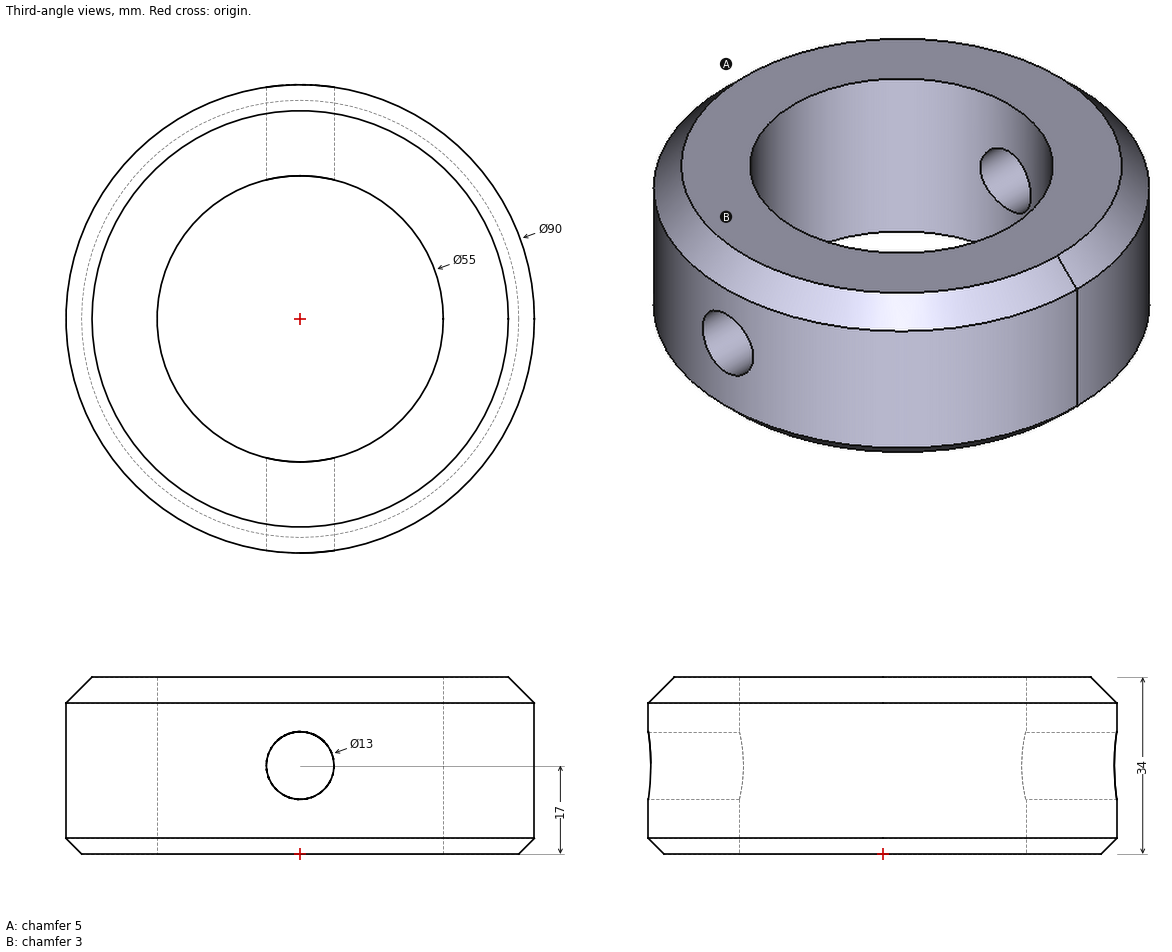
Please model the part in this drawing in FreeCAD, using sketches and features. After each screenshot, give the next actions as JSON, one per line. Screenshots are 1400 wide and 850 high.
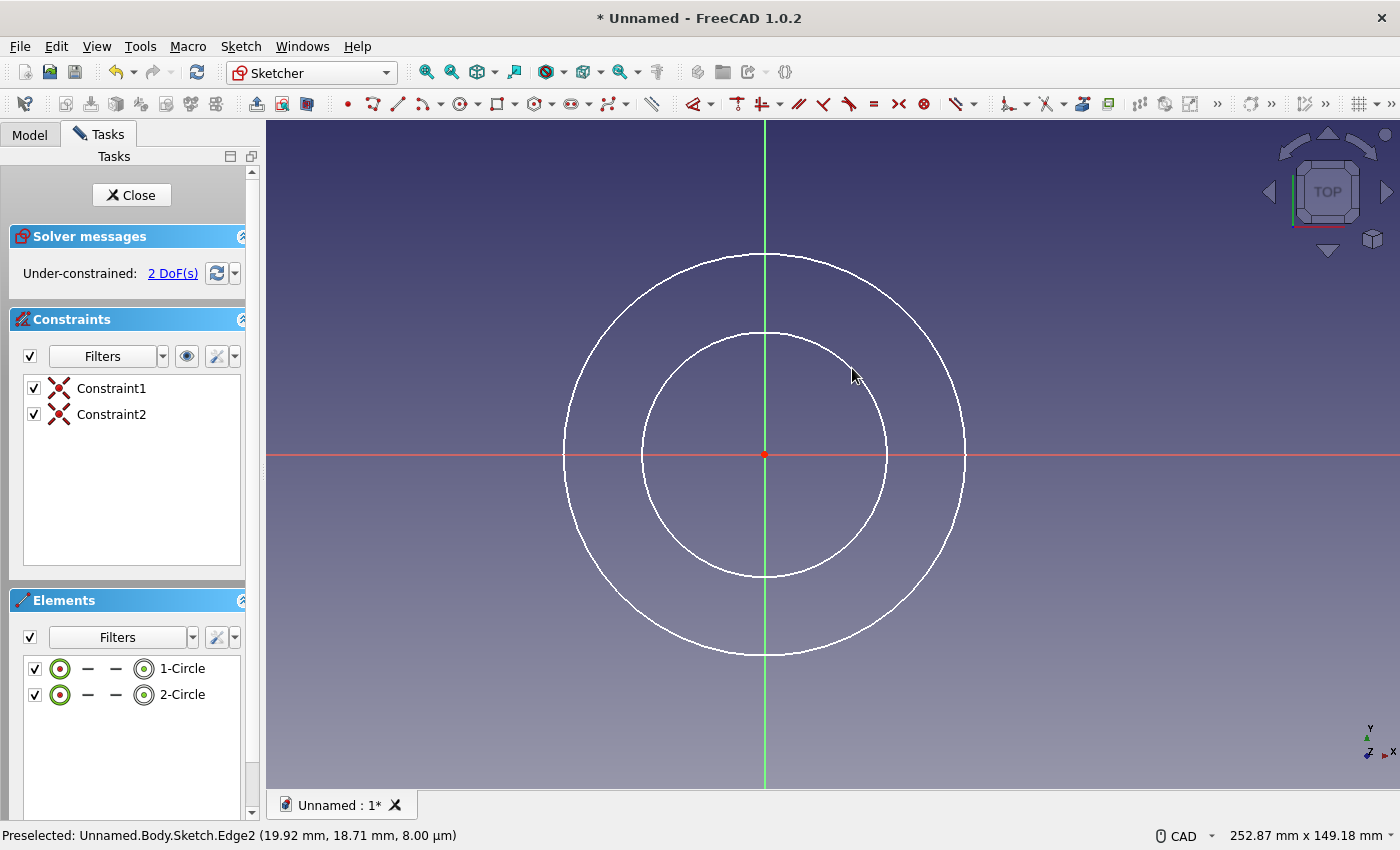
{"action": "left_click", "coordinate": [692, 104]}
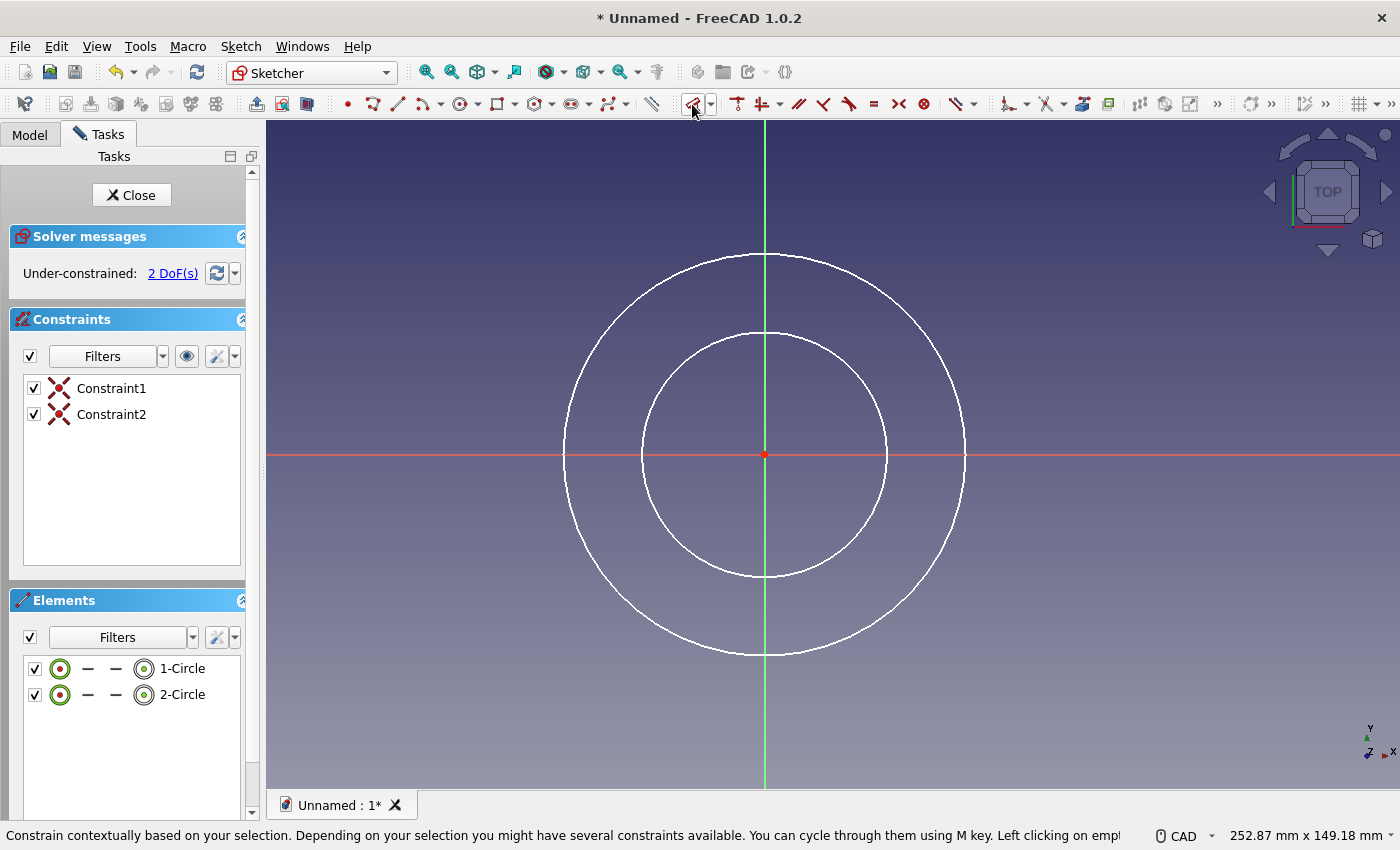
{"action": "left_click", "coordinate": [906, 312]}
{"action": "left_click", "coordinate": [929, 289]}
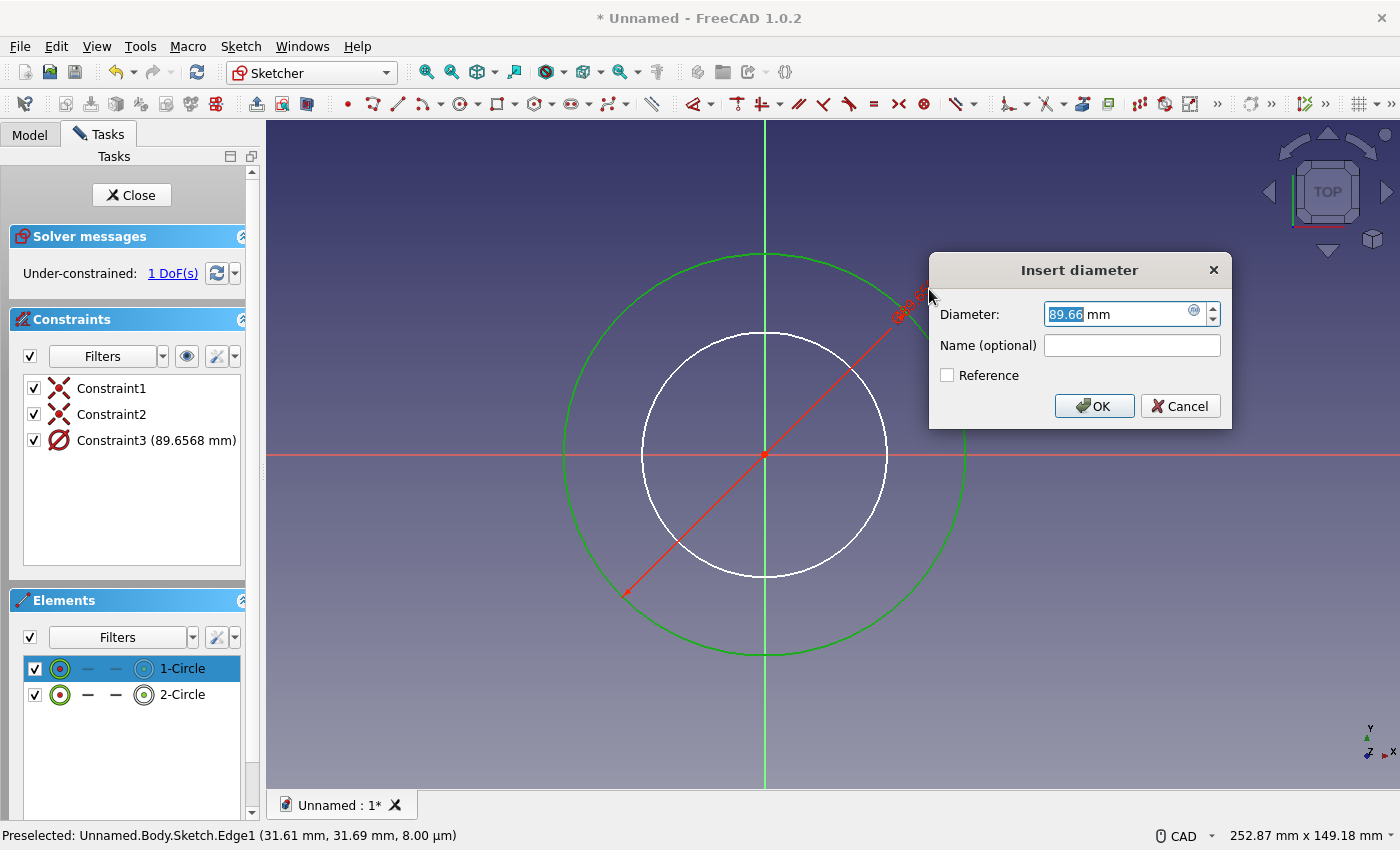
{"action": "type", "text": "90"}
{"action": "key", "text": "Return"}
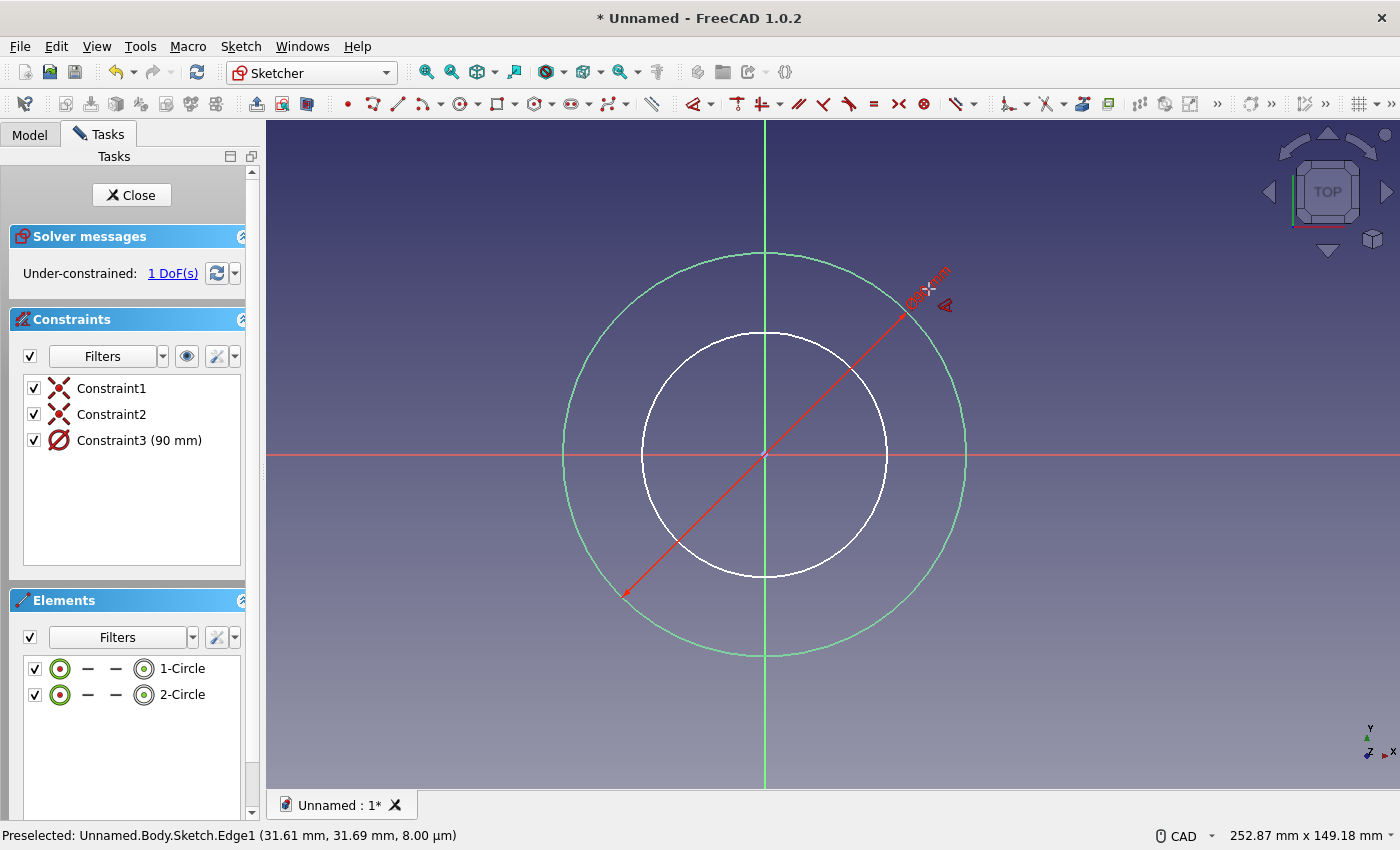
{"action": "left_click", "coordinate": [851, 368]}
{"action": "left_click", "coordinate": [874, 345]}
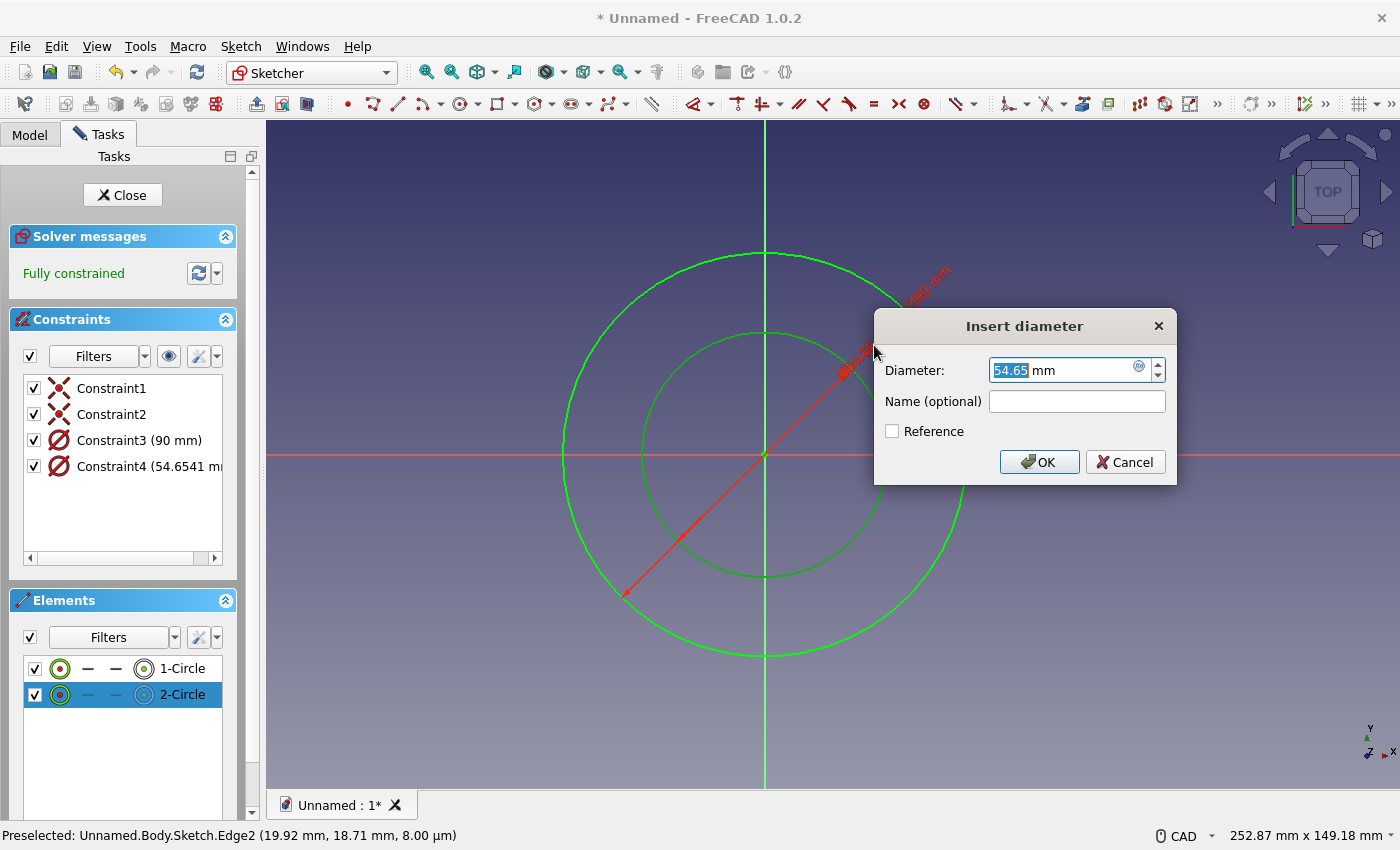
{"action": "type", "text": "55"}
{"action": "key", "text": "Return"}
{"action": "key", "text": "Escape"}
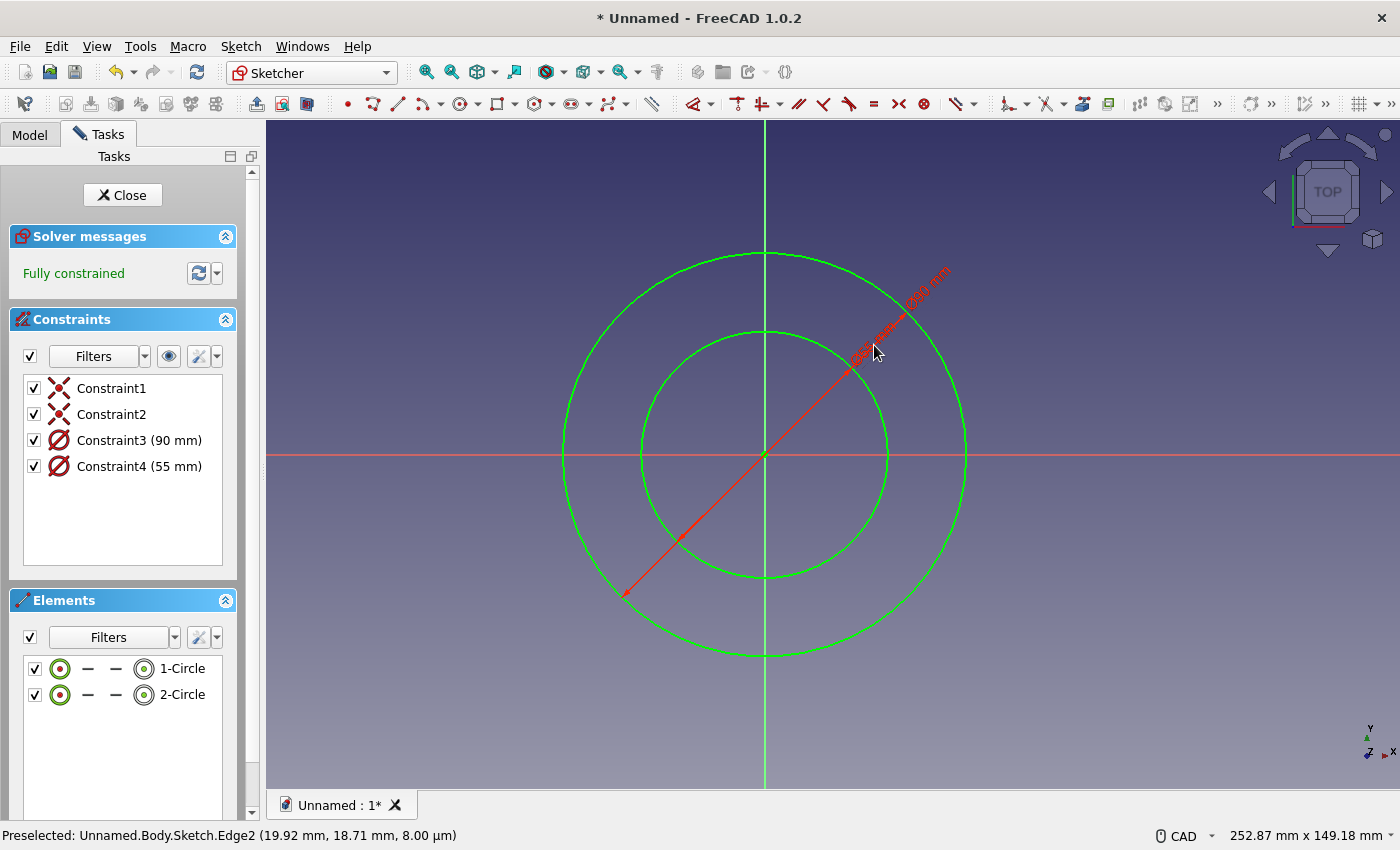
{"action": "left_click", "coordinate": [123, 195]}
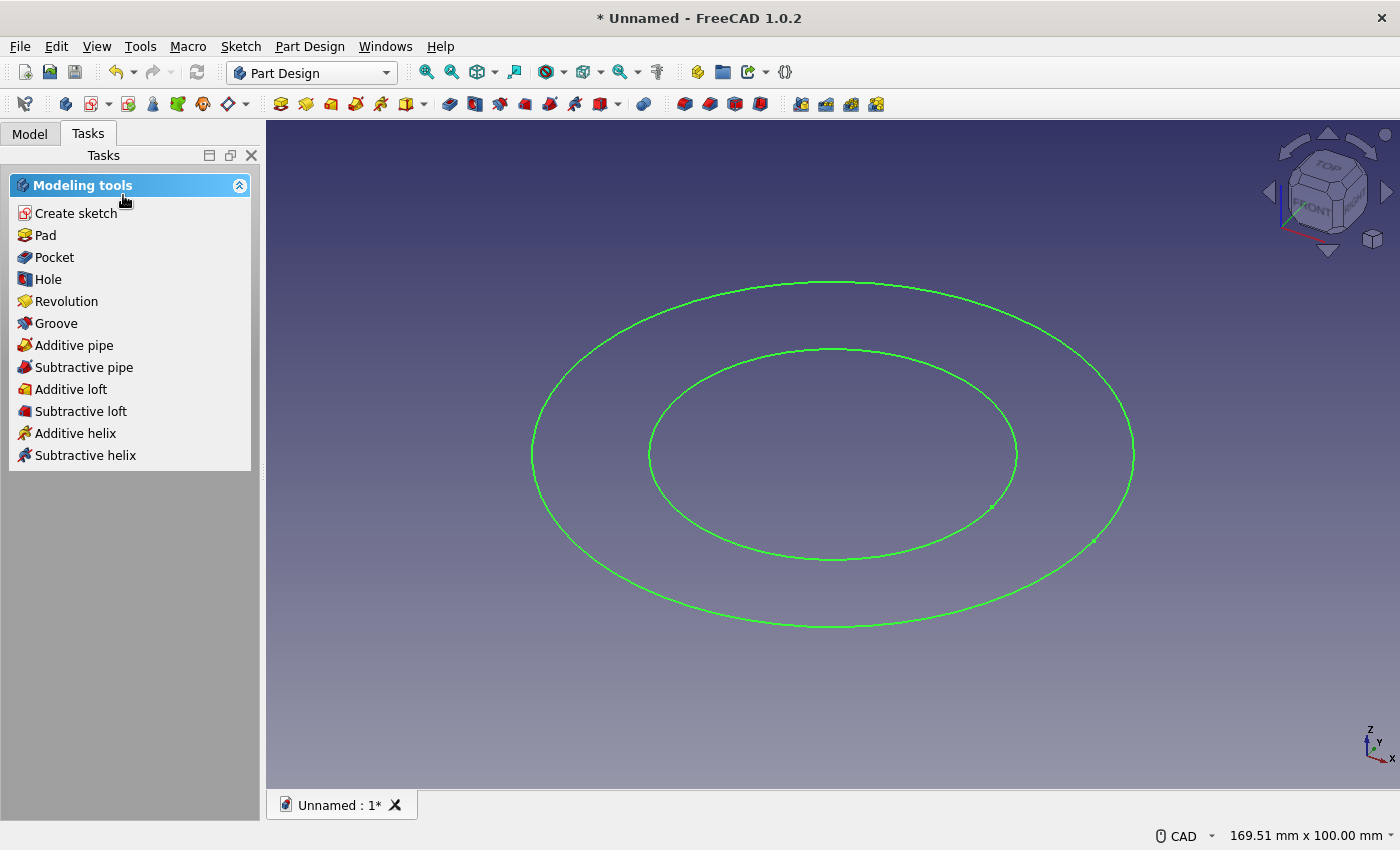
{"action": "left_click", "coordinate": [281, 104]}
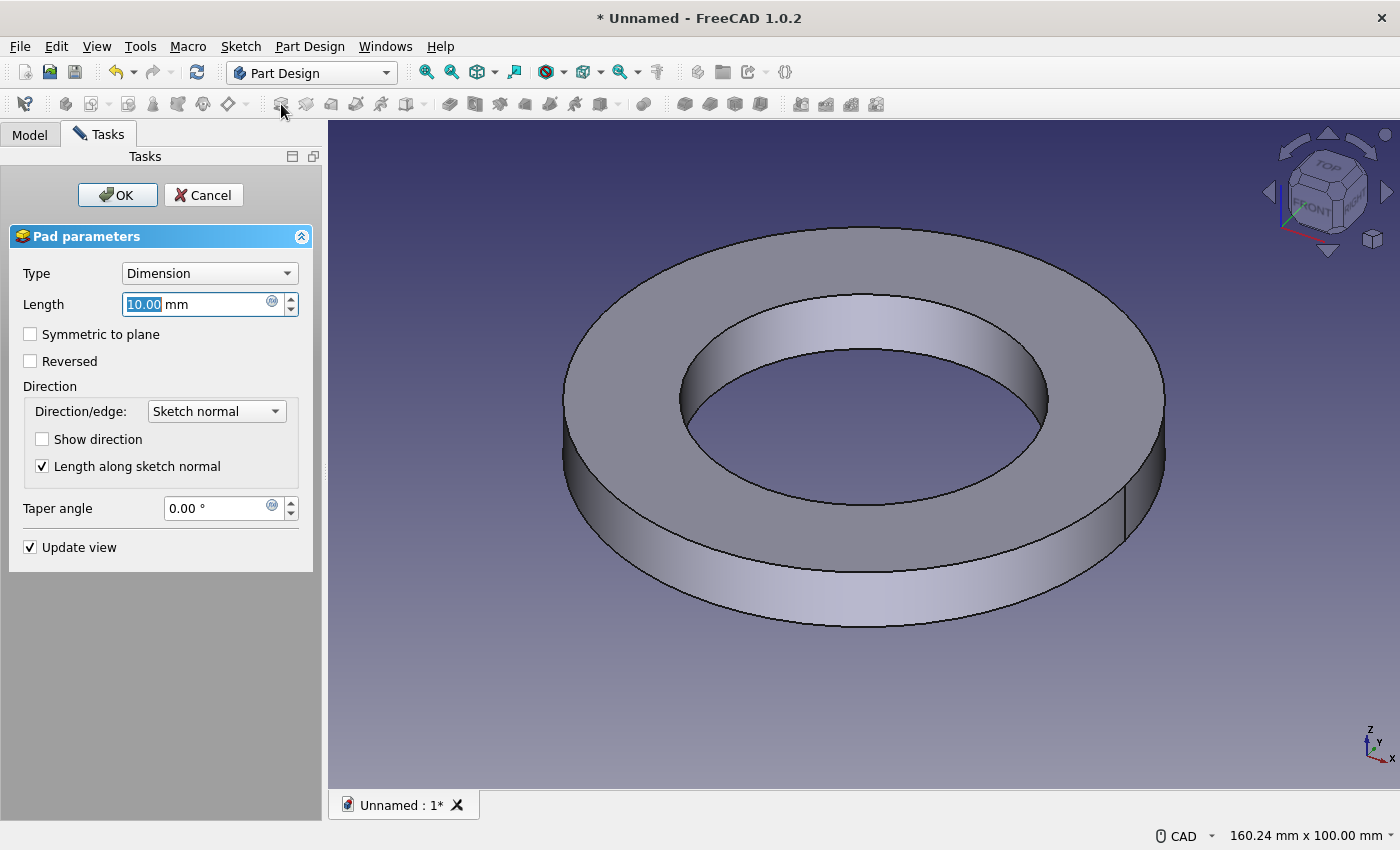
{"action": "type", "text": "34"}
{"action": "key", "text": "Tab"}